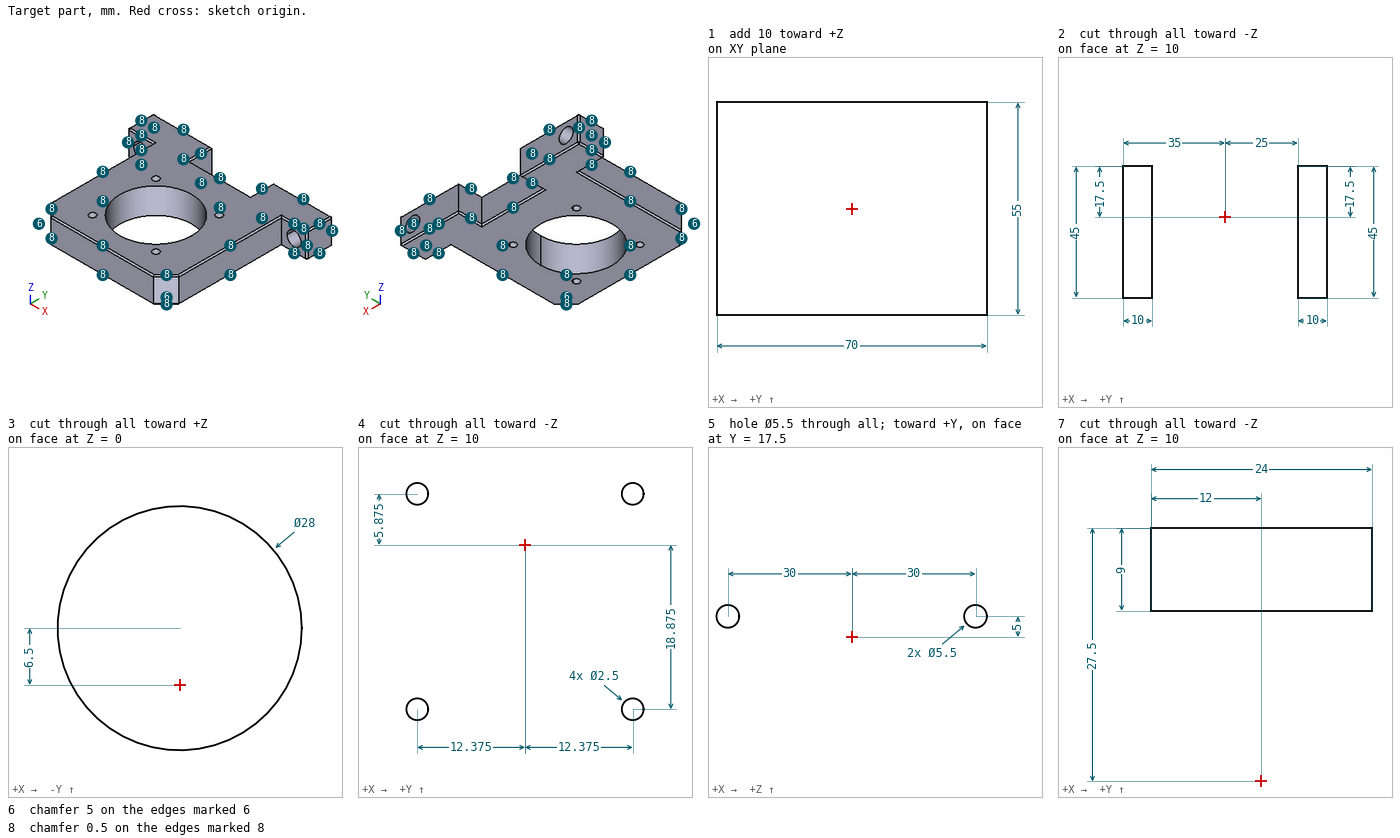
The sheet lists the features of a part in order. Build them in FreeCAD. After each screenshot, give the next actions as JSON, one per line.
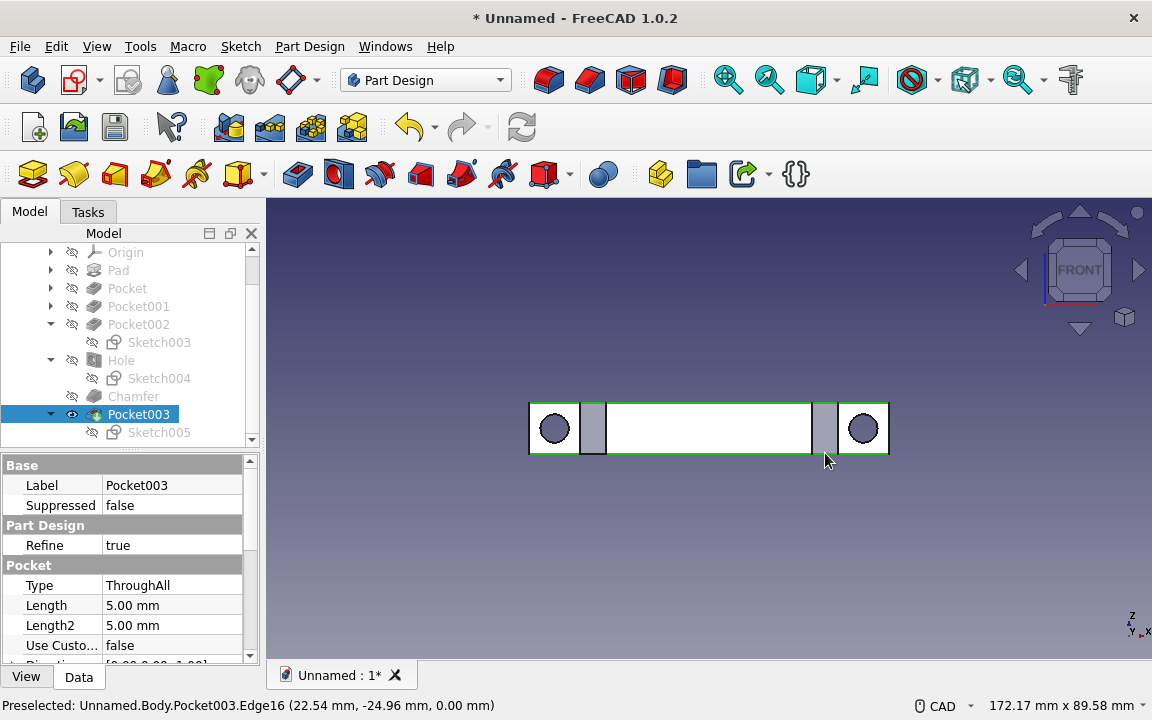
{"action": "left_click", "coordinate": [593, 453], "text": "ctrl"}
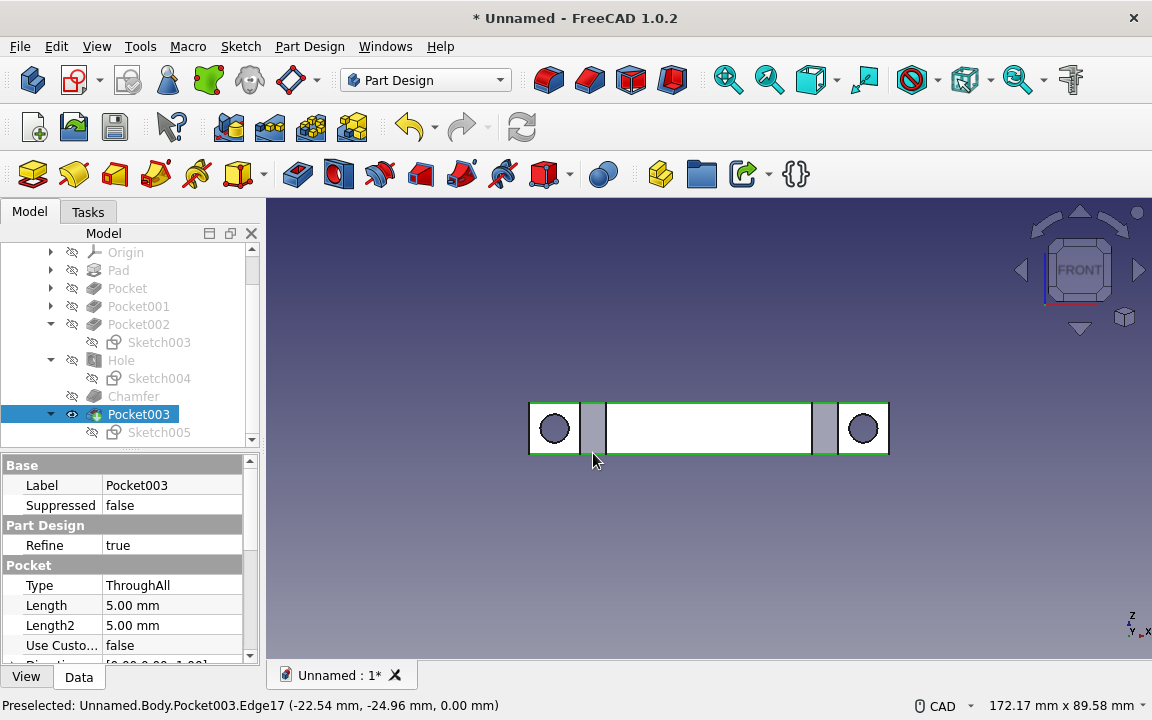
{"action": "key", "text": "3"}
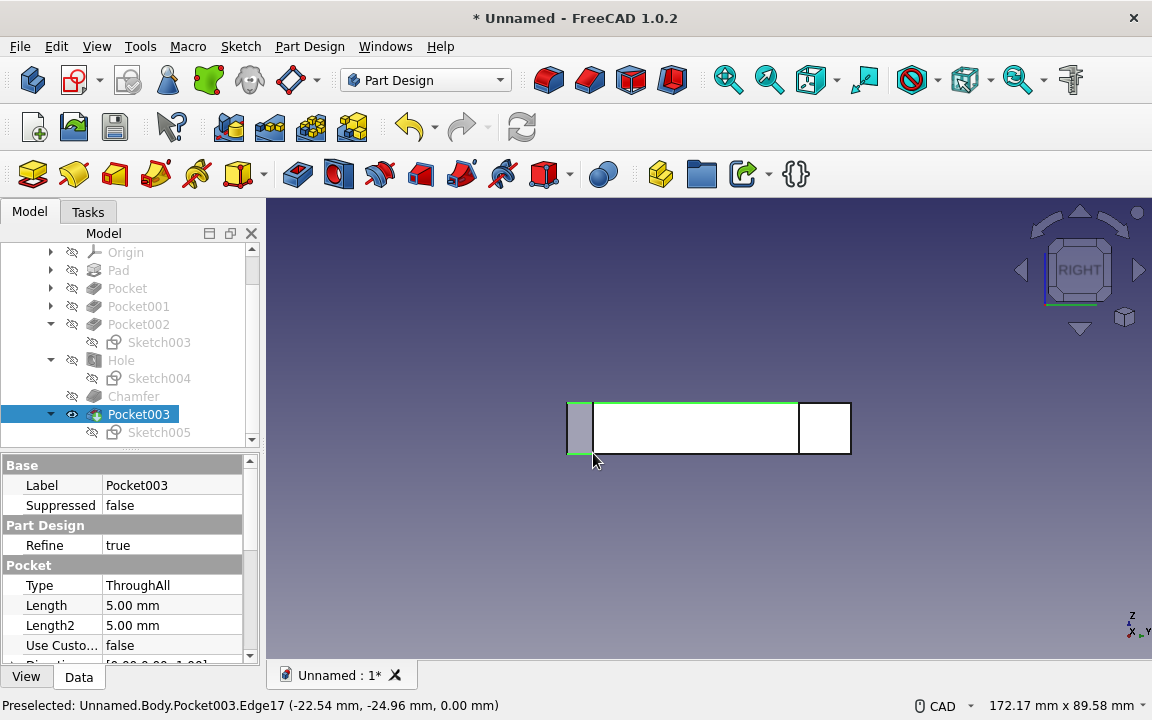
{"action": "left_click", "coordinate": [729, 80]}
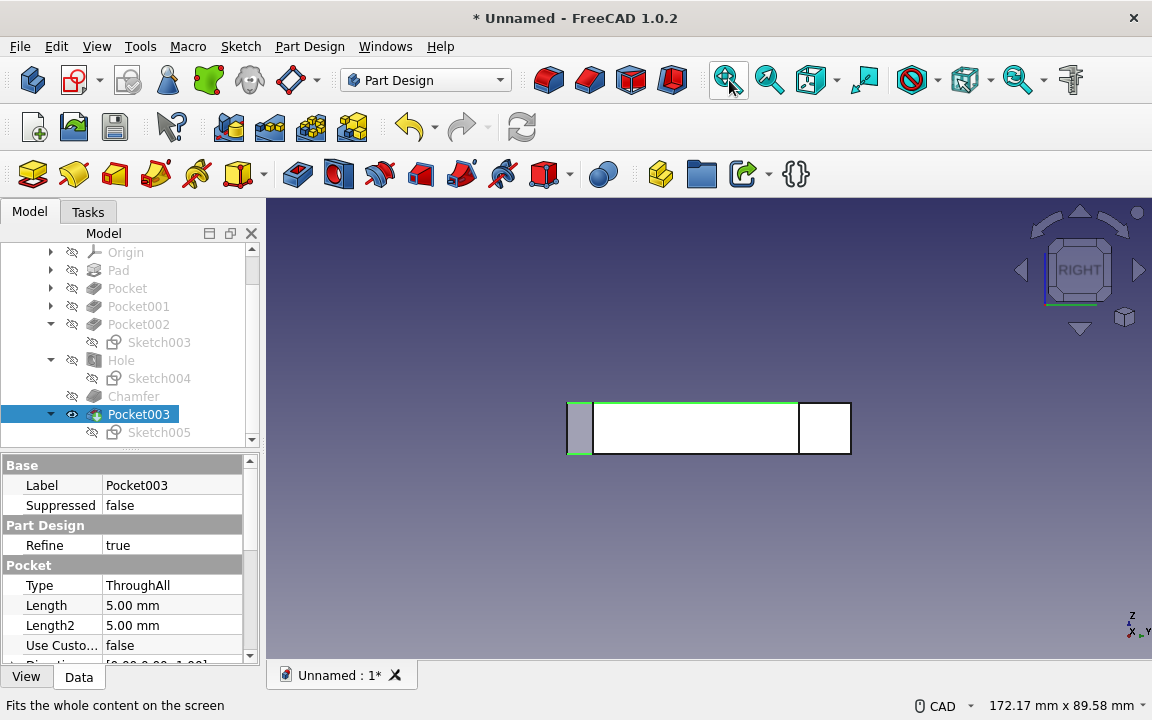
{"action": "left_click", "coordinate": [696, 453], "text": "ctrl"}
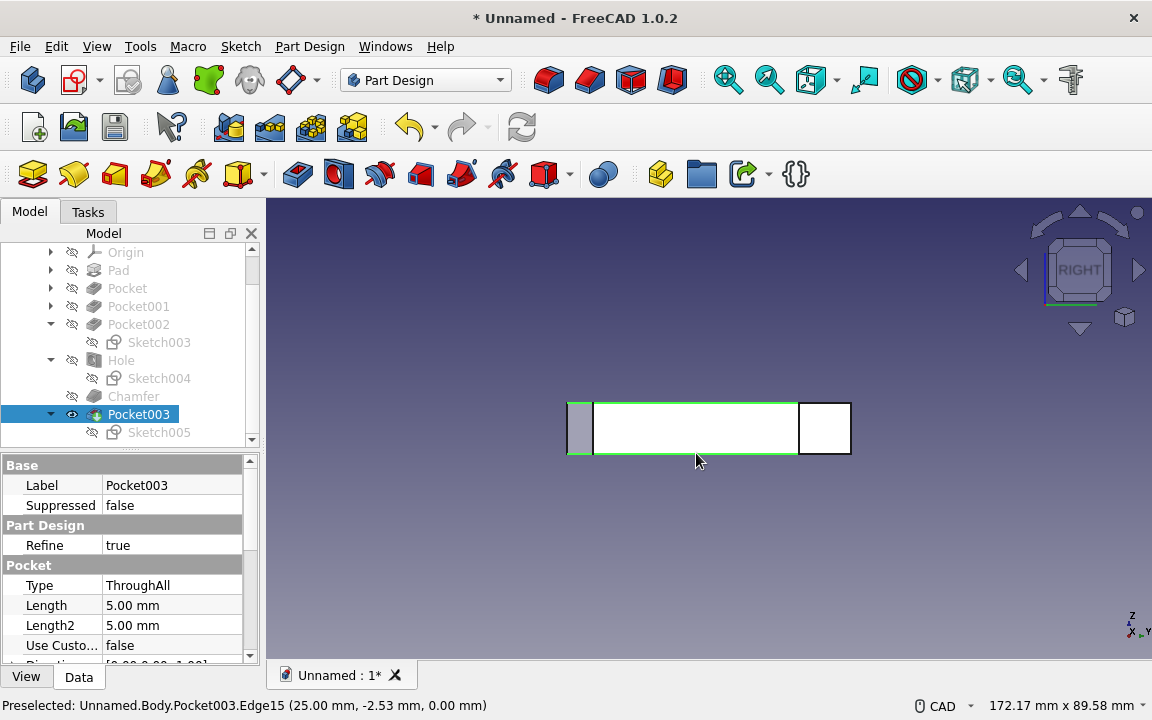
{"action": "key", "text": "5"}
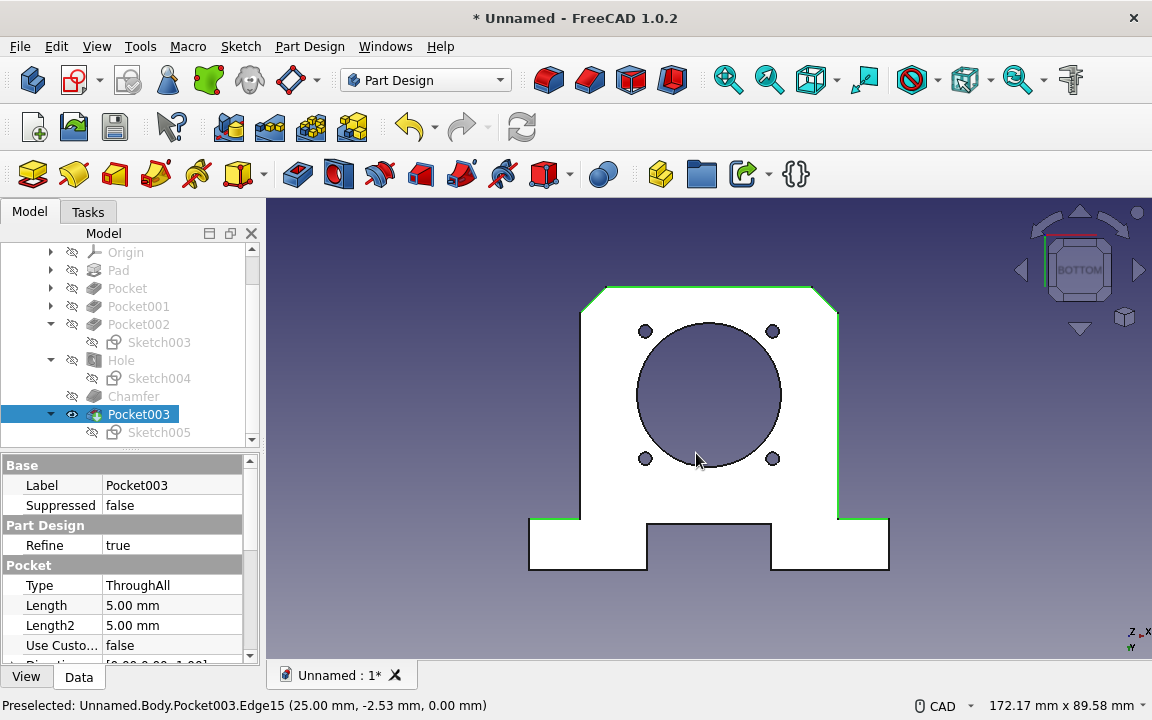
{"action": "left_click", "coordinate": [830, 569], "text": "ctrl"}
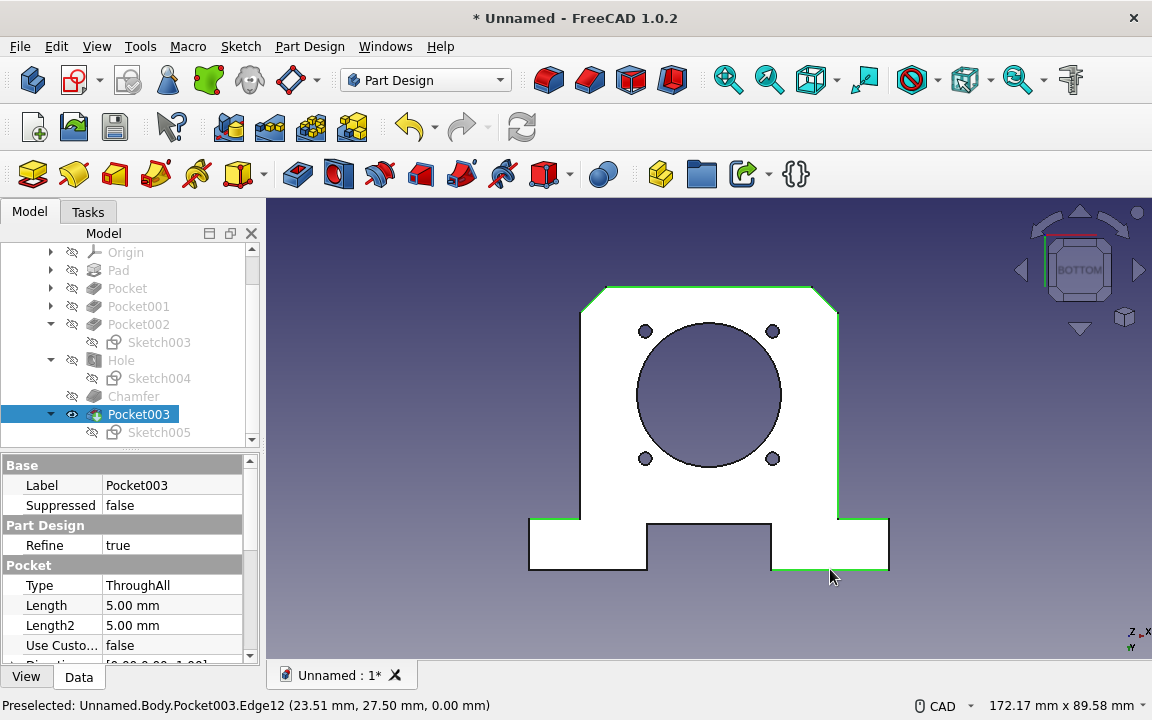
{"action": "left_click", "coordinate": [580, 415], "text": "ctrl"}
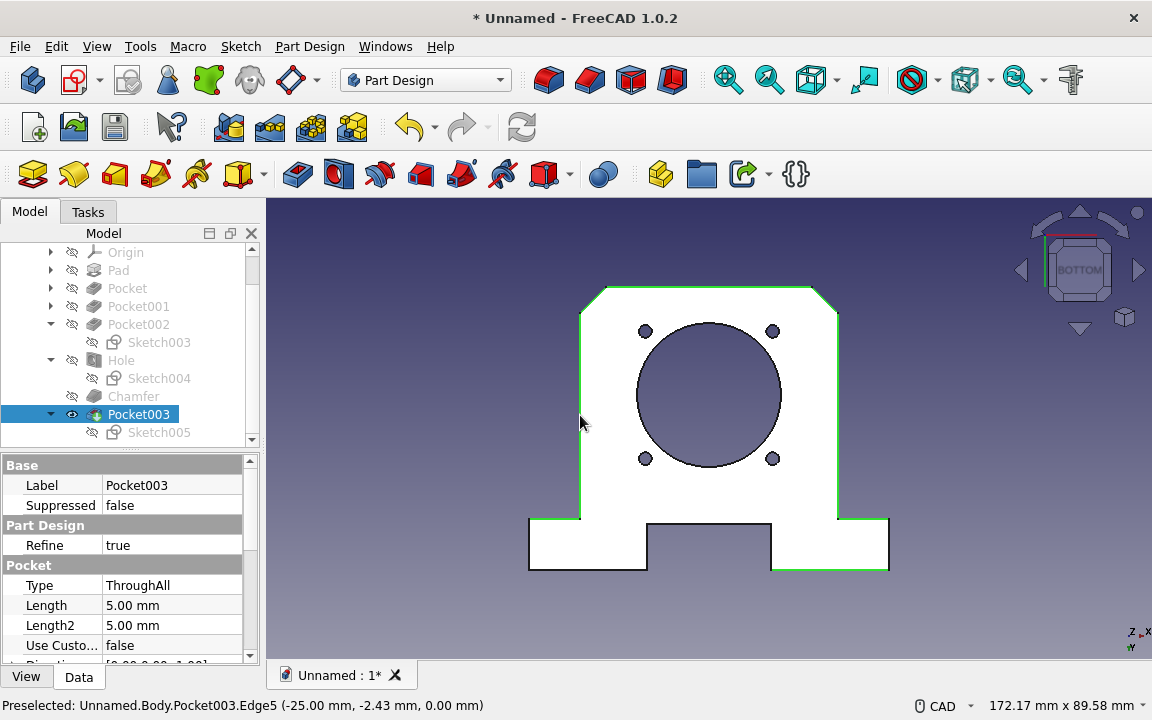
{"action": "left_click", "coordinate": [588, 569], "text": "ctrl"}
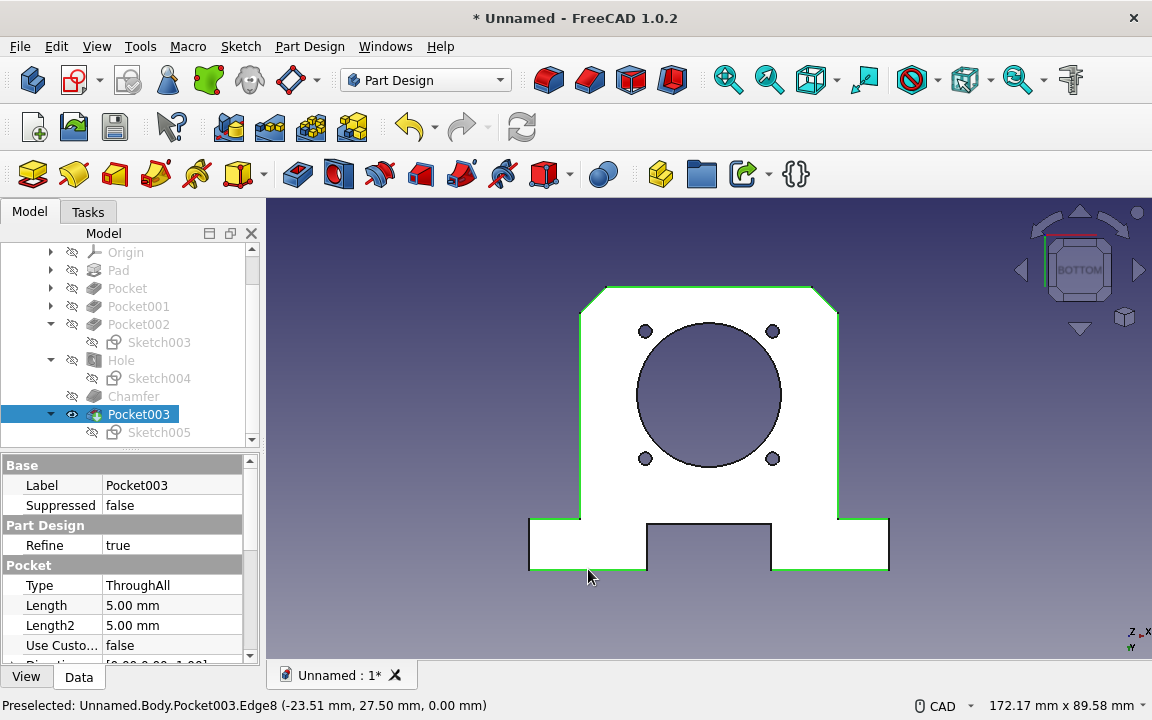
{"action": "left_click", "coordinate": [647, 546], "text": "ctrl"}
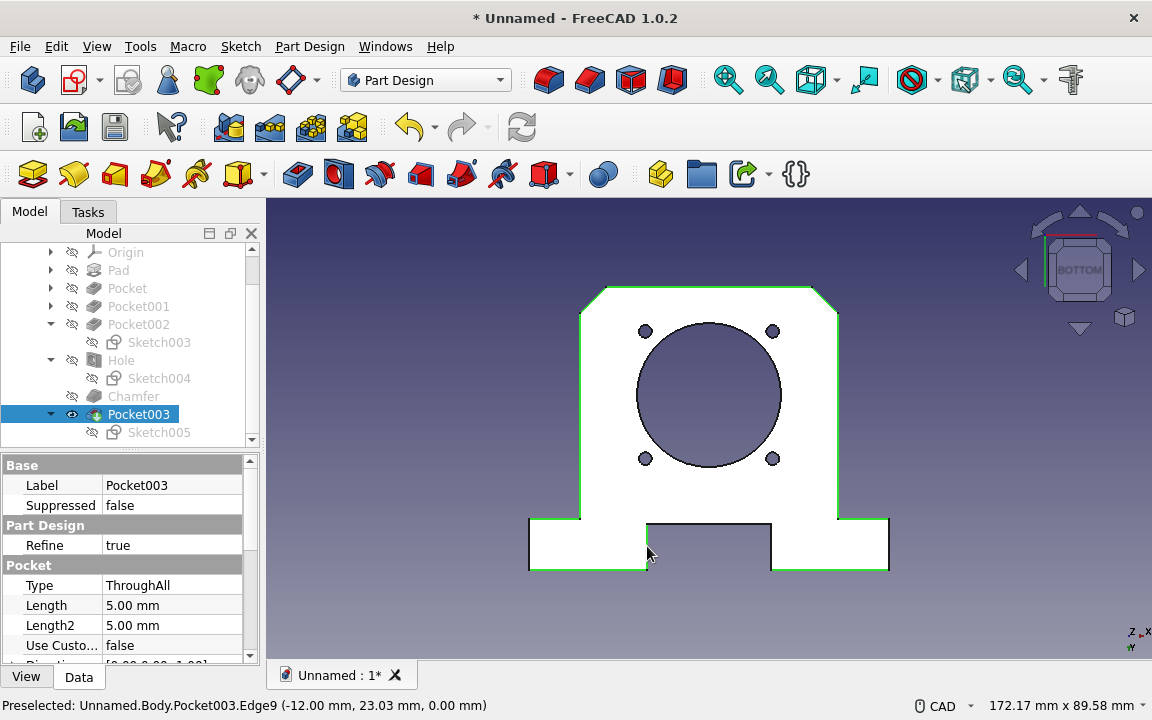
{"action": "left_click", "coordinate": [771, 546], "text": "ctrl"}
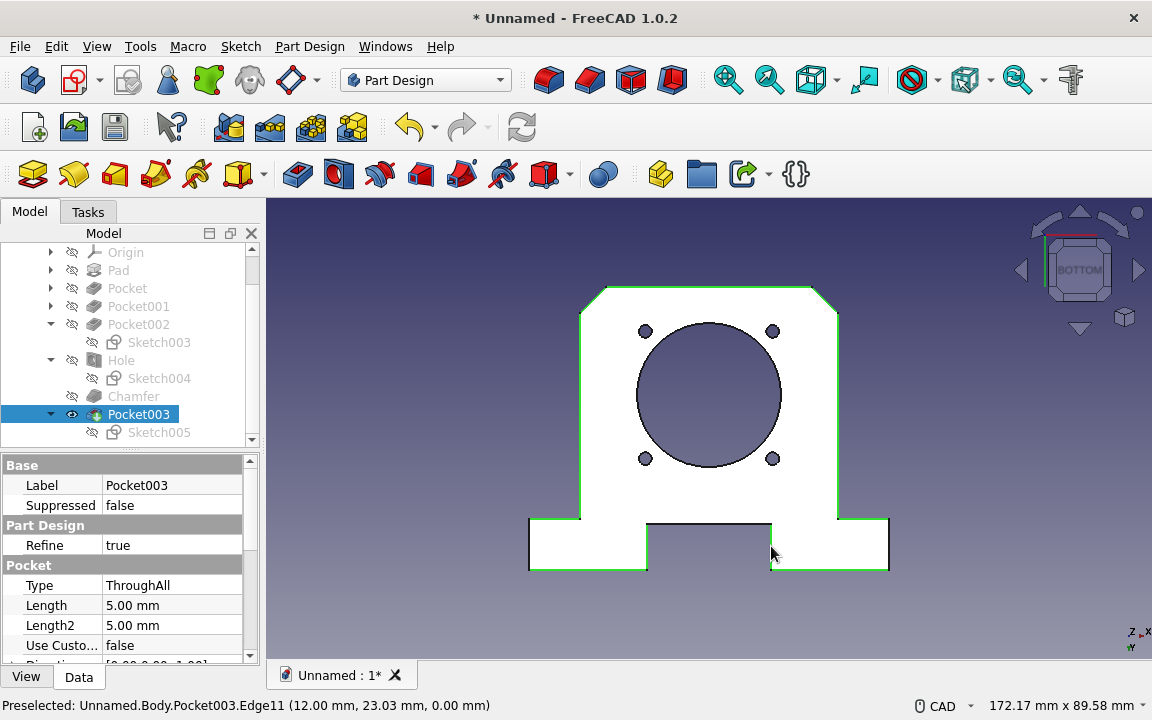
{"action": "left_click", "coordinate": [709, 523], "text": "ctrl"}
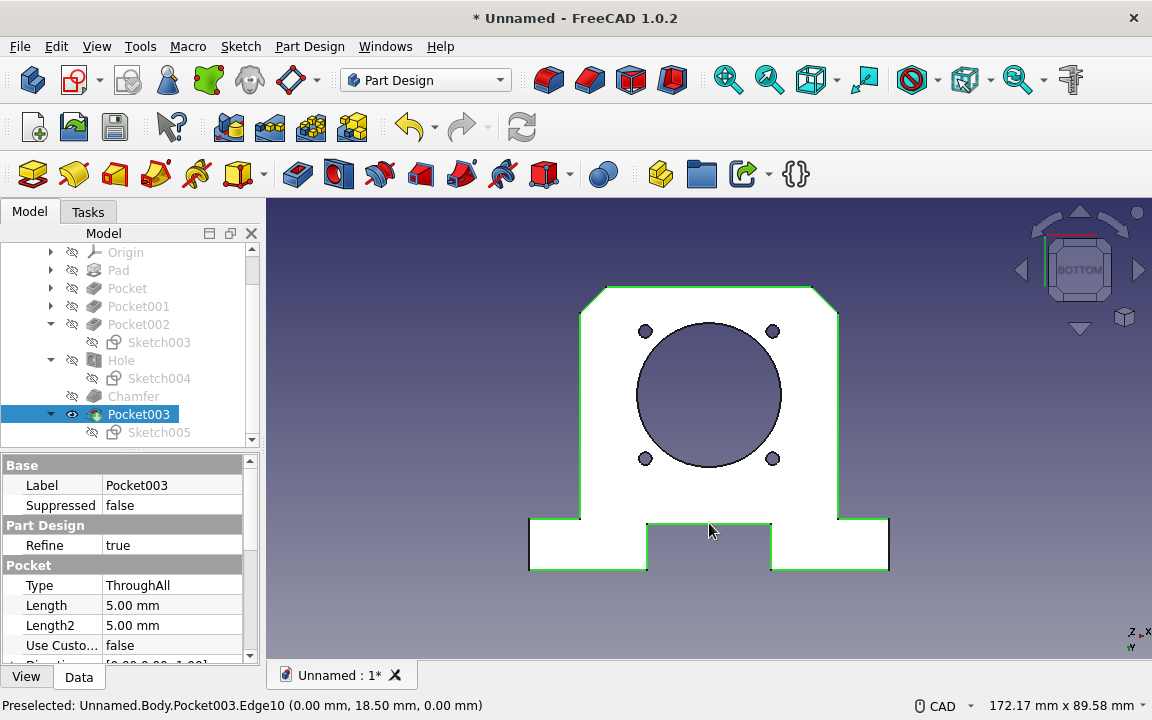
{"action": "key", "text": "4"}